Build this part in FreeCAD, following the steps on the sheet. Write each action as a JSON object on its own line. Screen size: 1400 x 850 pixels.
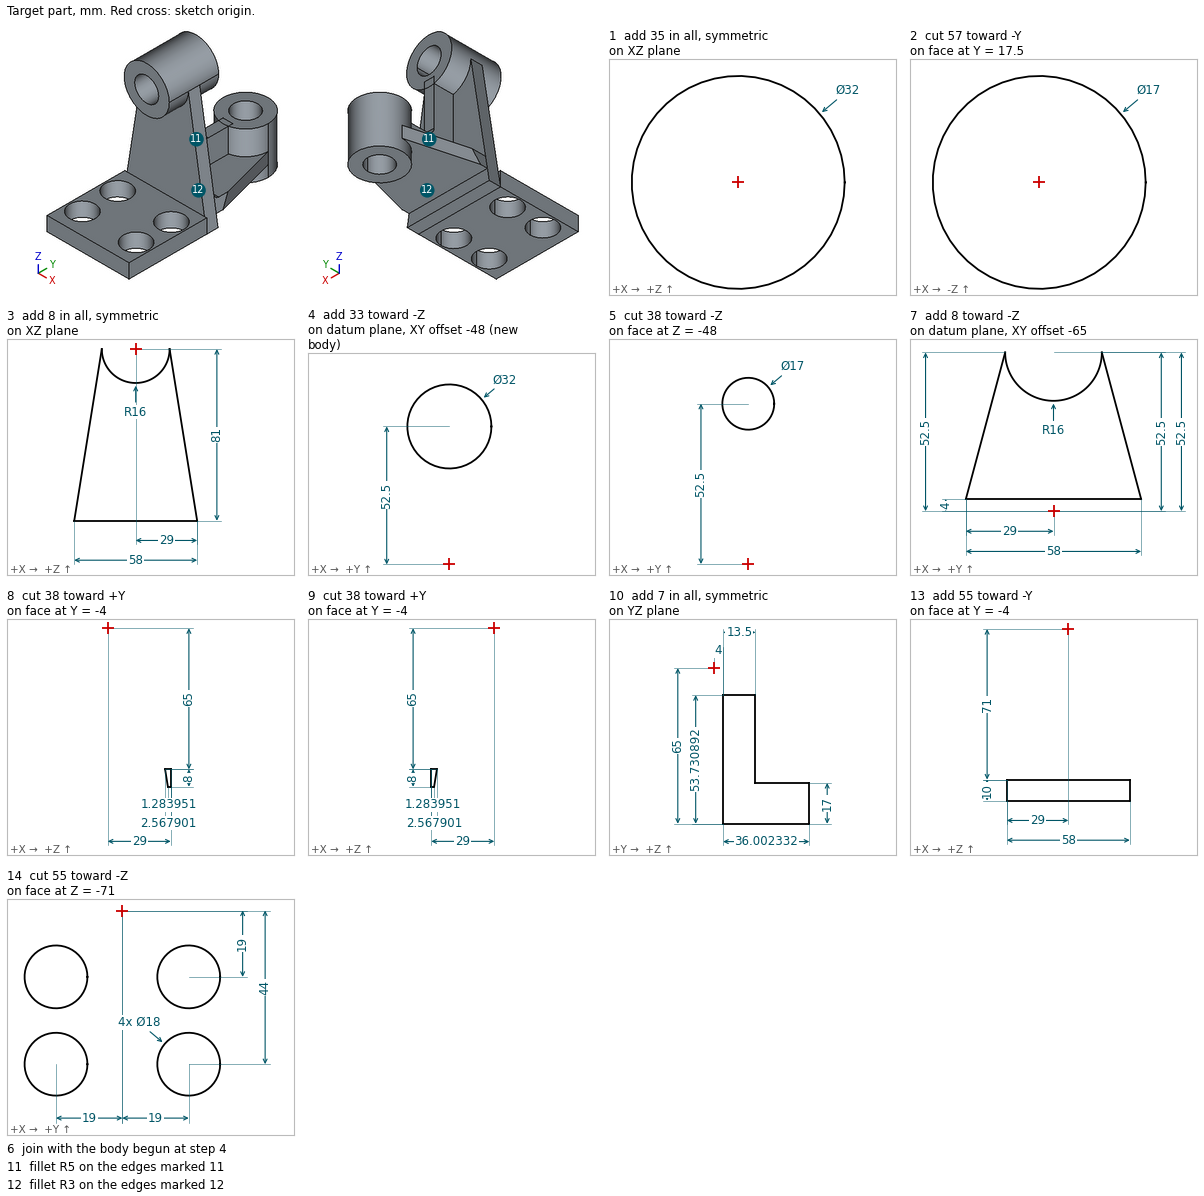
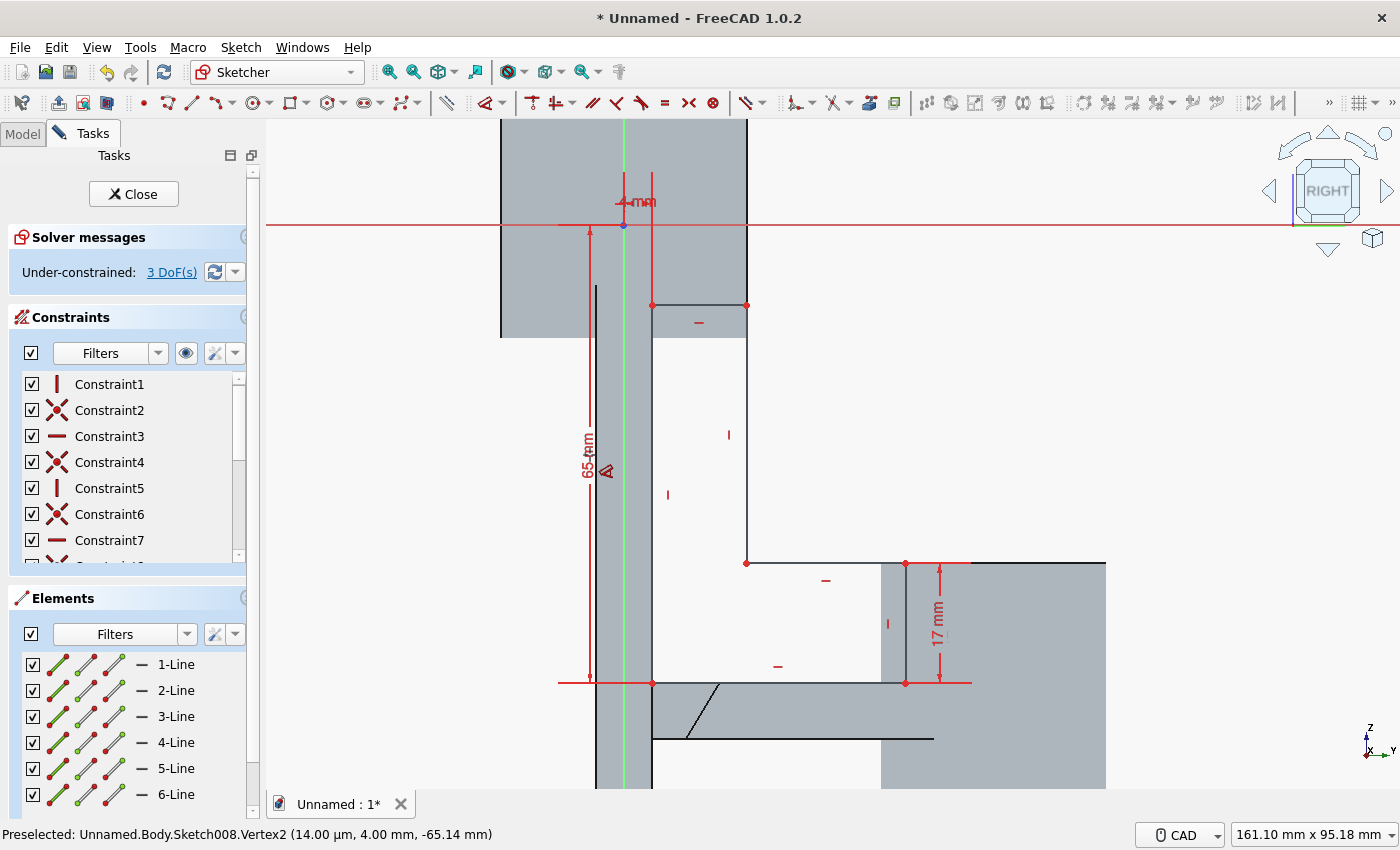
{"action": "left_click", "coordinate": [718, 305]}
{"action": "left_click", "coordinate": [699, 271]}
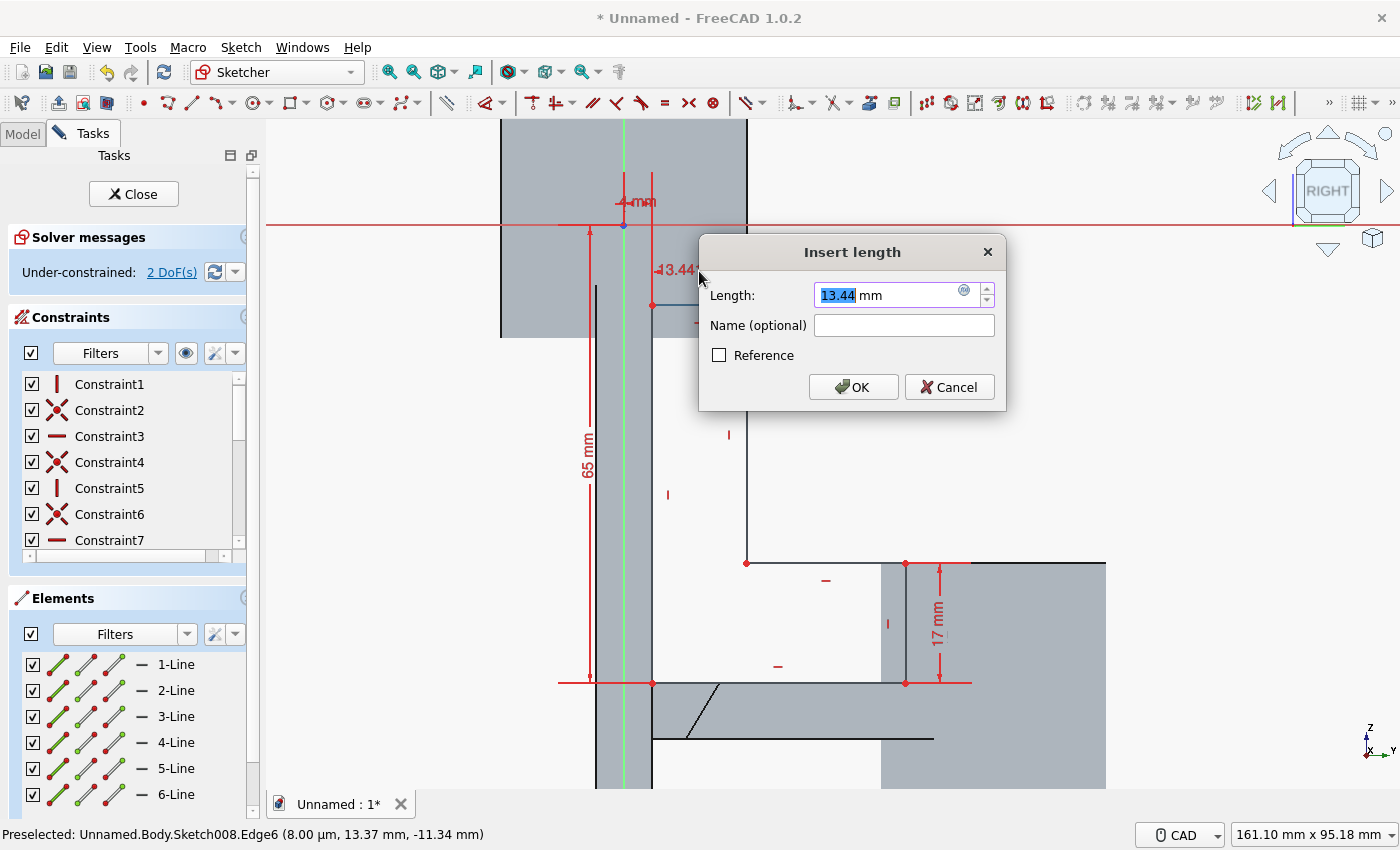
{"action": "type", "text": "13.5"}
{"action": "key", "text": "Return"}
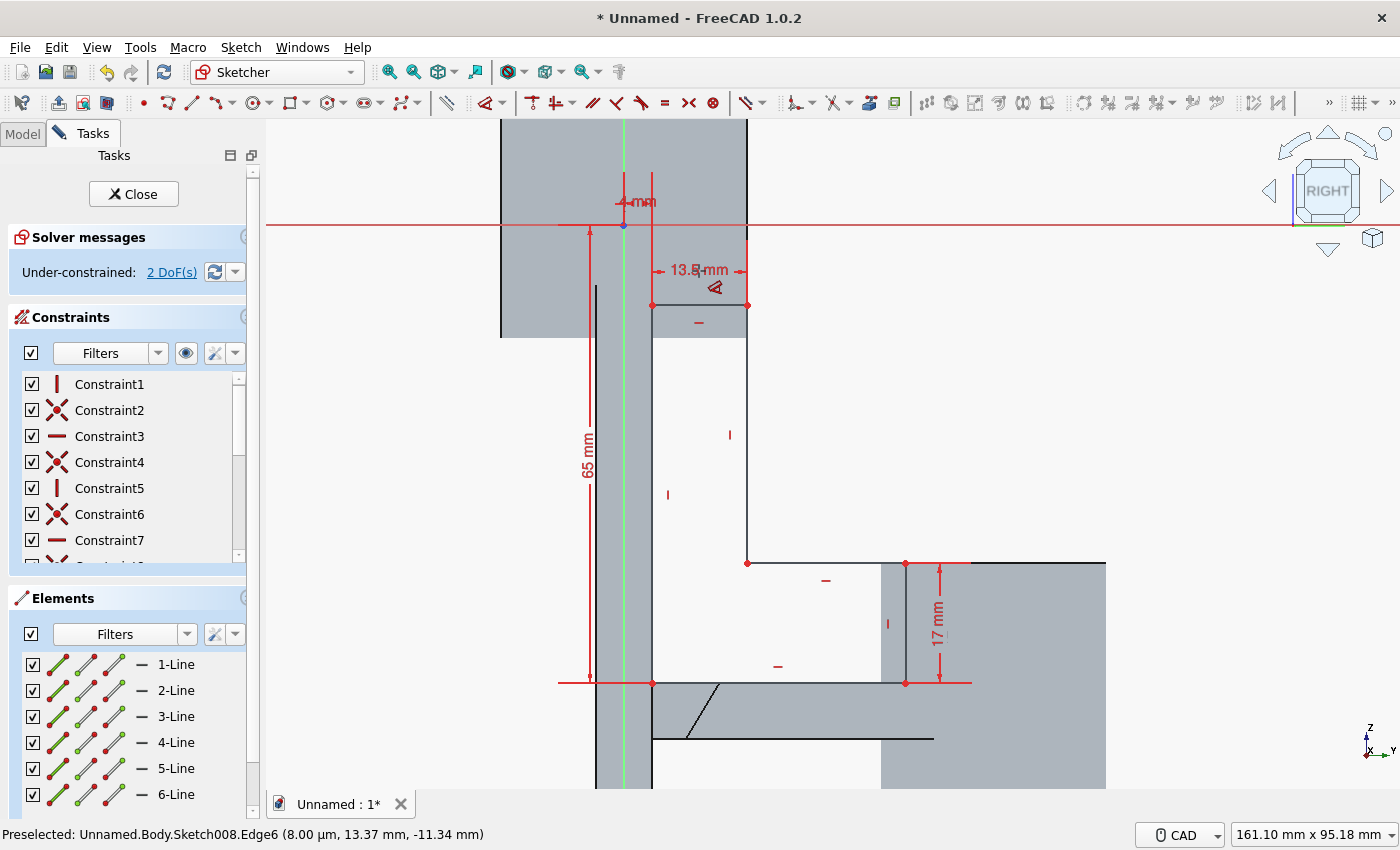
{"action": "left_click", "coordinate": [652, 419]}
{"action": "left_click", "coordinate": [686, 494]}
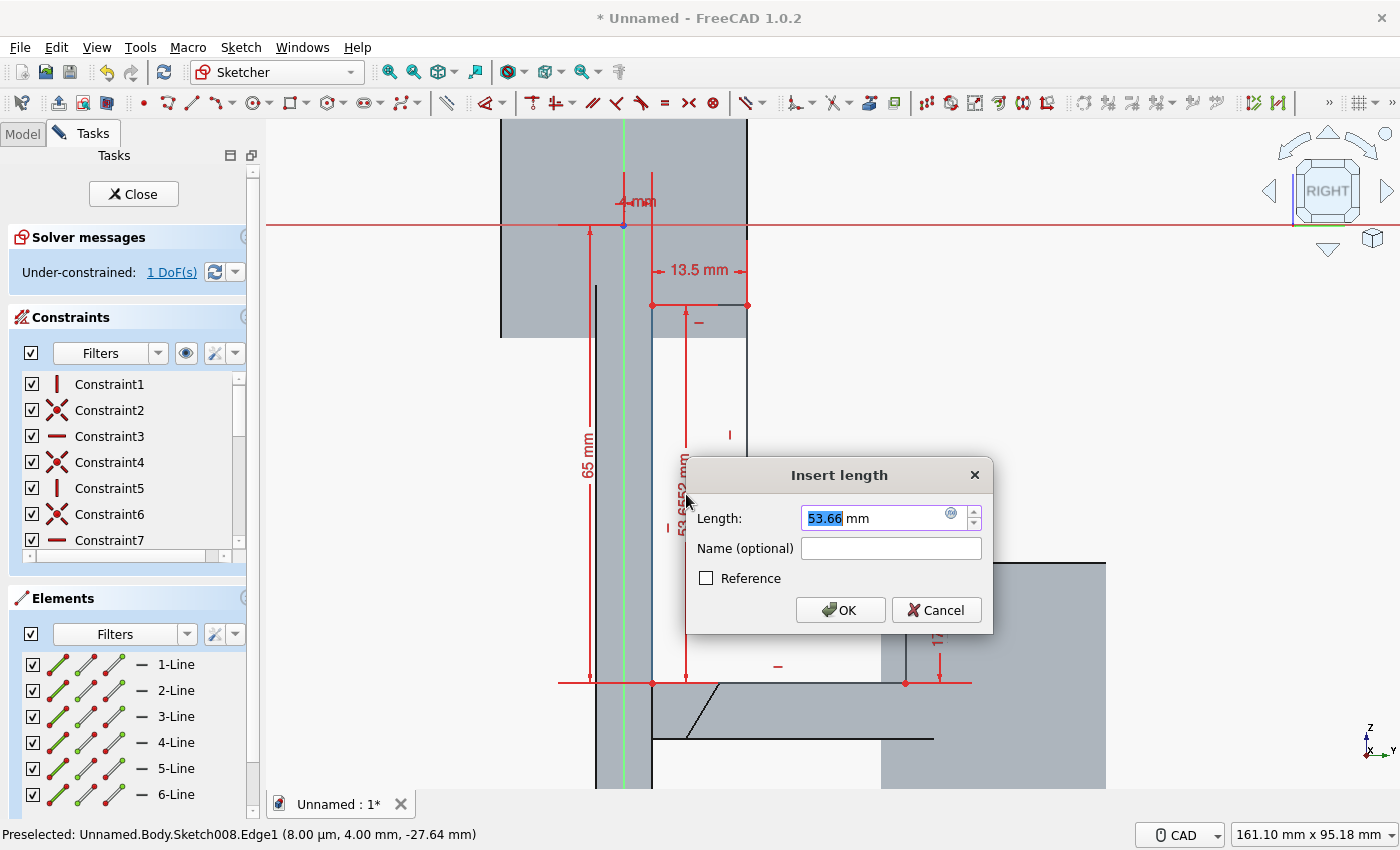
{"action": "type", "text": "53.730892"}
{"action": "key", "text": "Return"}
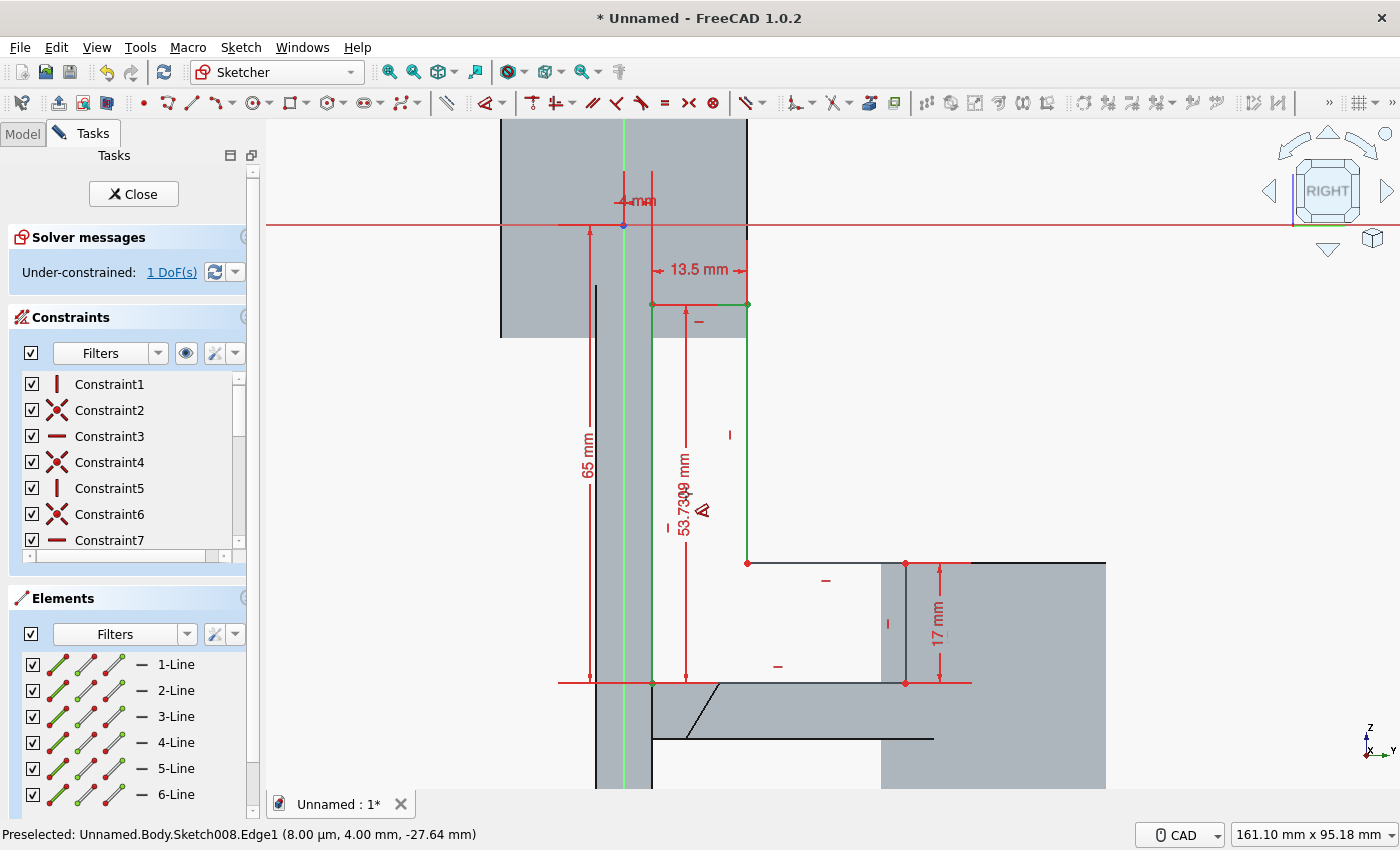
{"action": "left_click", "coordinate": [728, 683]}
{"action": "left_click", "coordinate": [779, 717]}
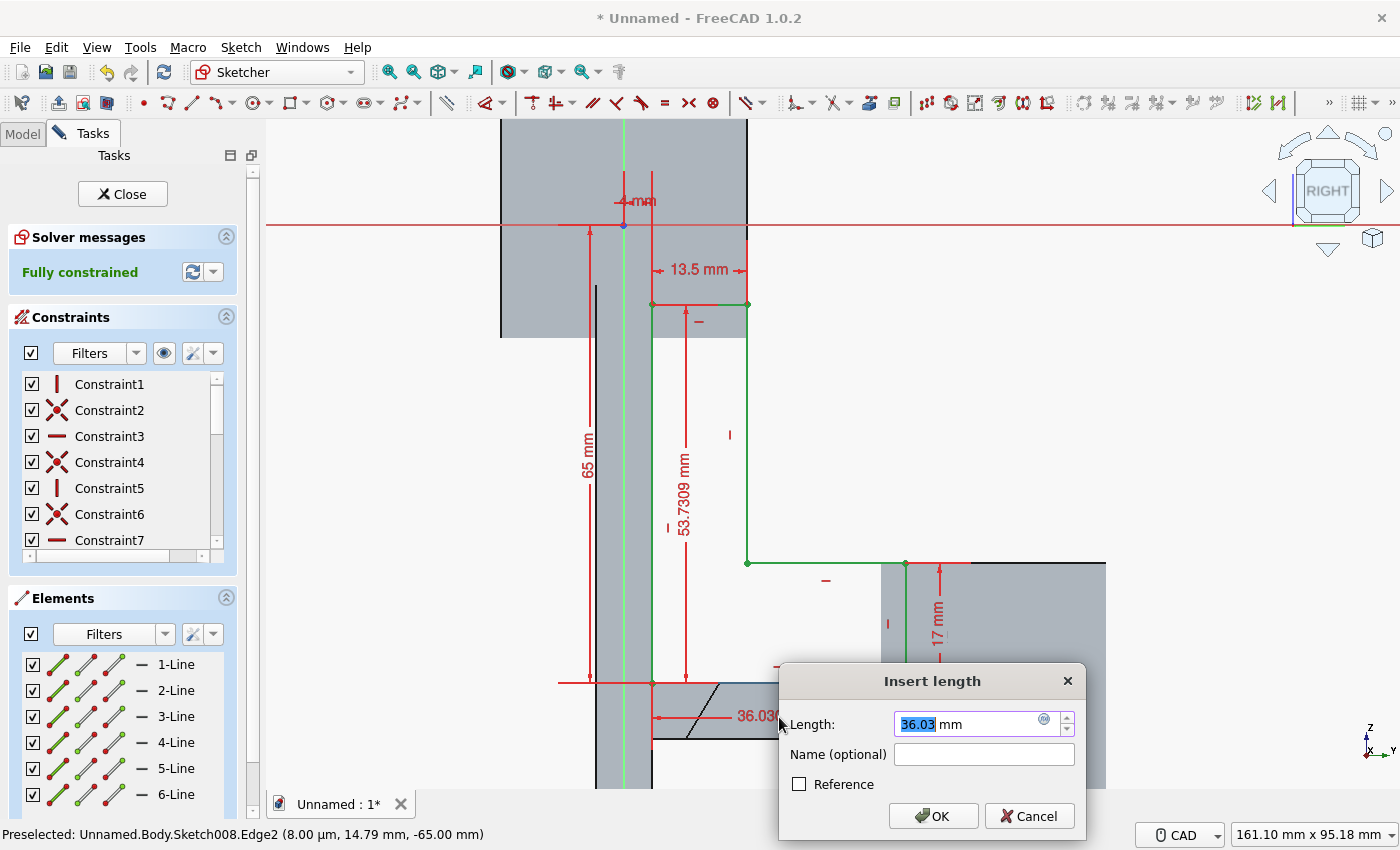
{"action": "type", "text": "36.002332"}
{"action": "key", "text": "Return"}
{"action": "key", "text": "Escape"}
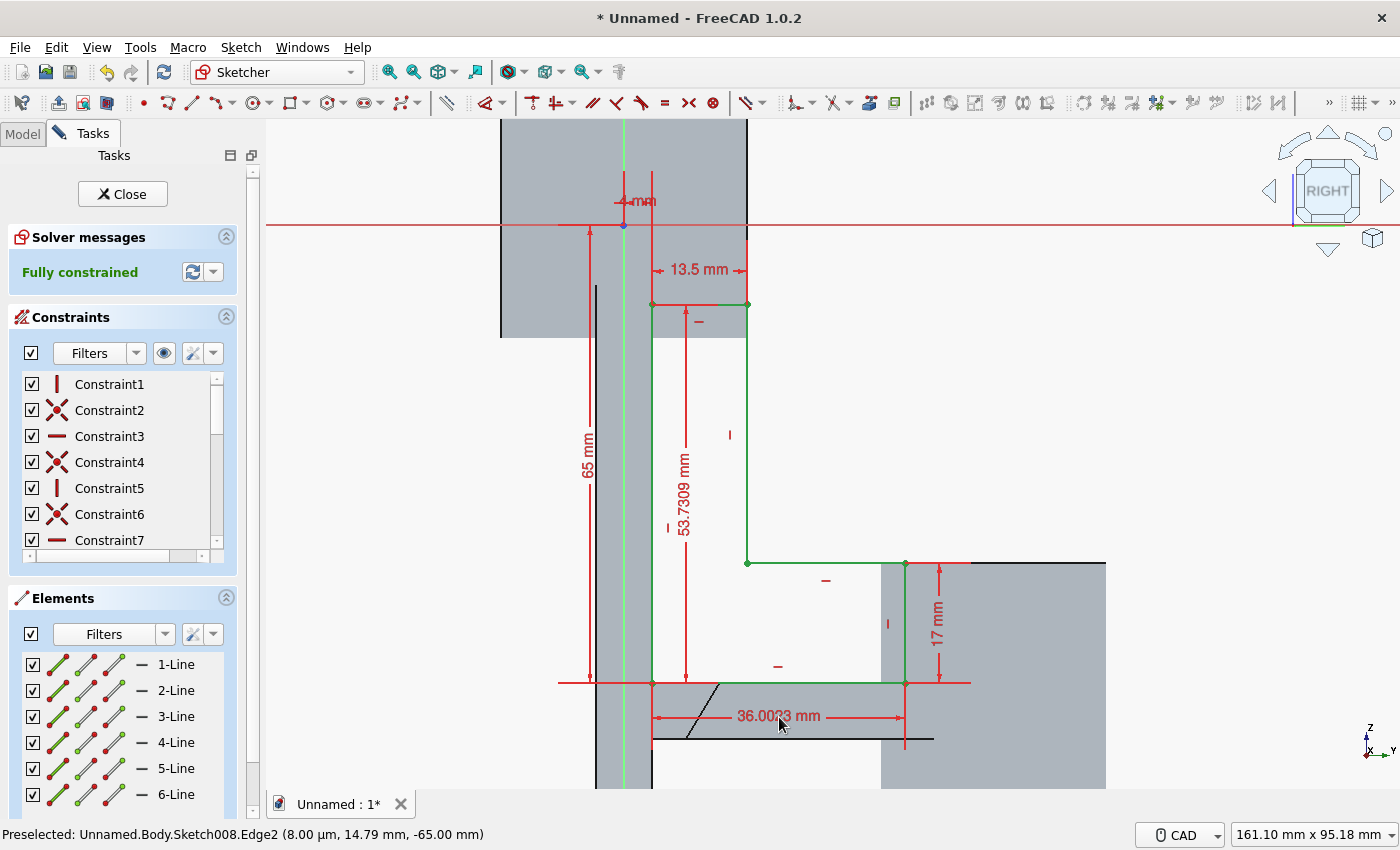
{"action": "left_click", "coordinate": [123, 194]}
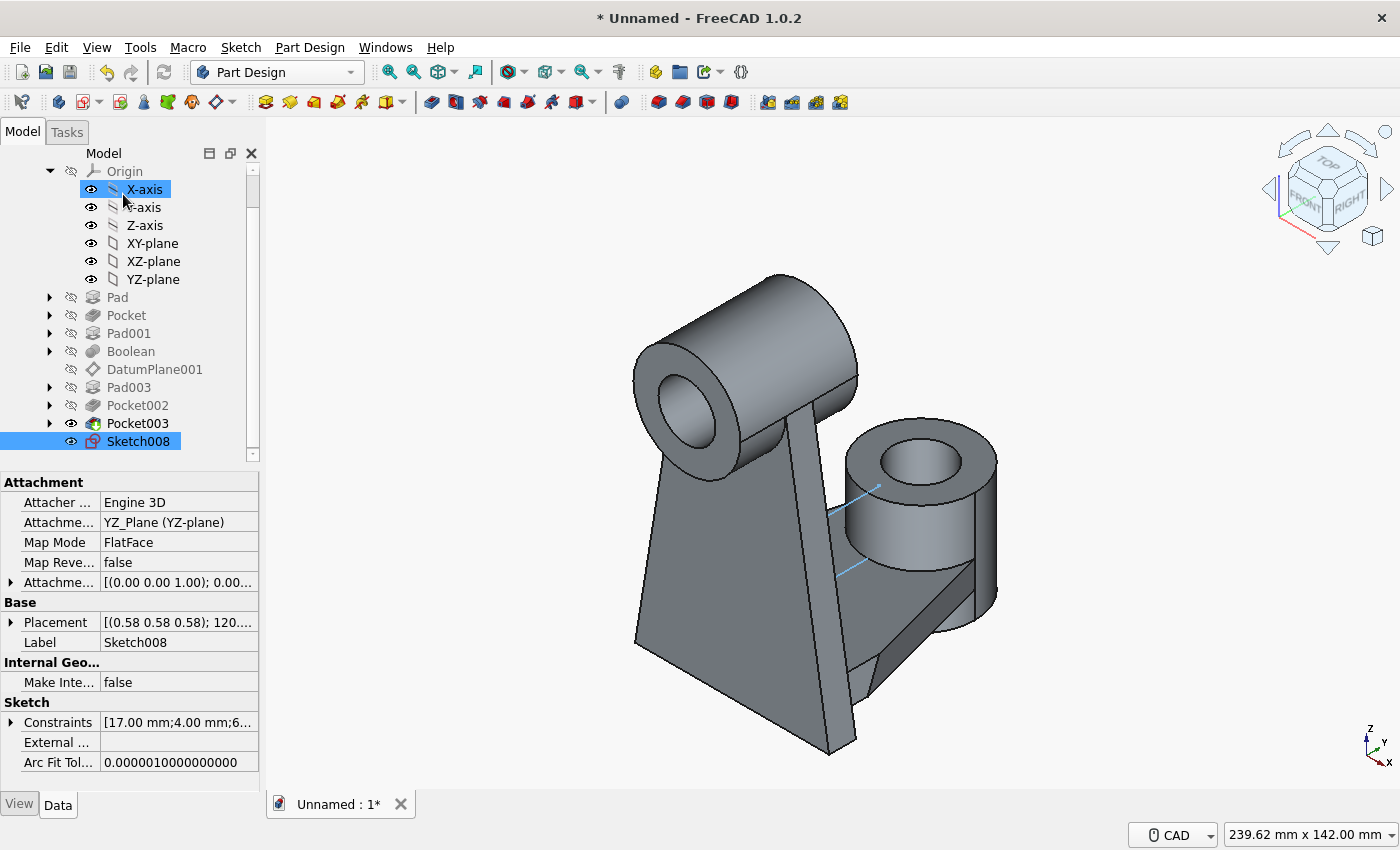
{"action": "left_click", "coordinate": [266, 102]}